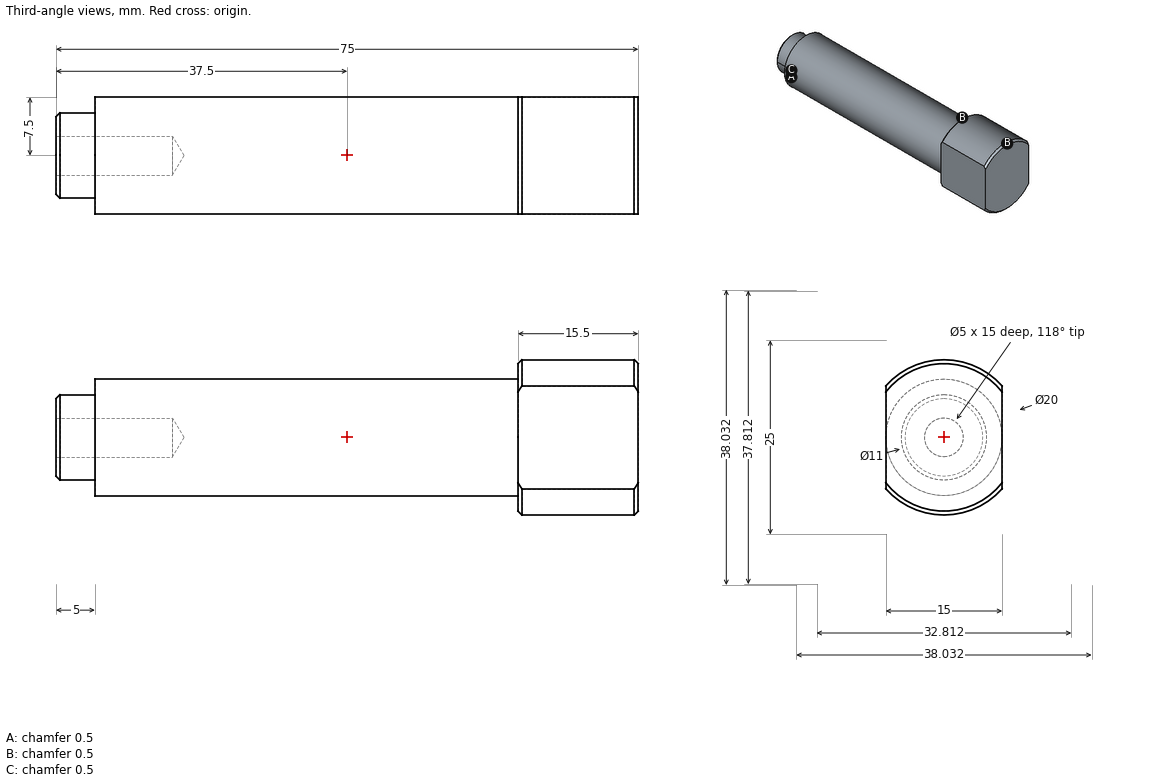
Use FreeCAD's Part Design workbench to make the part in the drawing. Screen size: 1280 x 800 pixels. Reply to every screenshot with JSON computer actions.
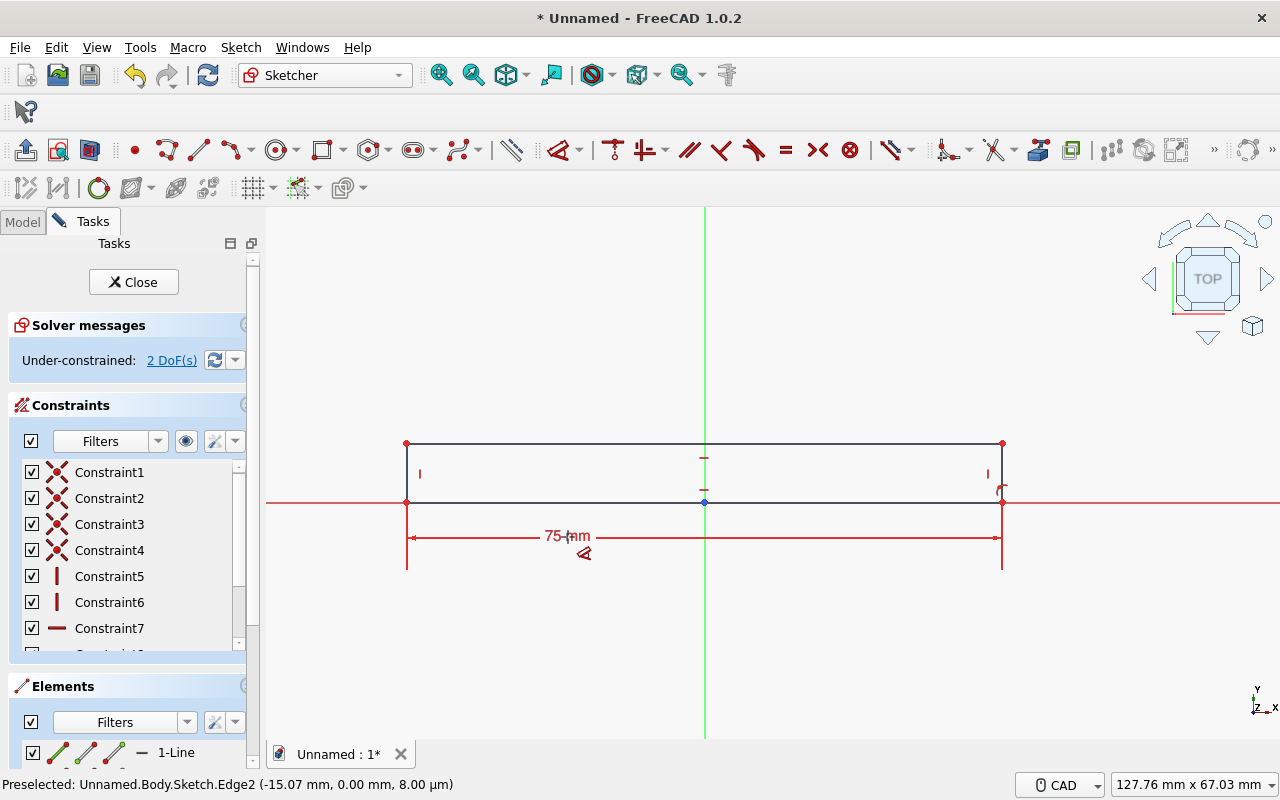
{"action": "left_click", "coordinate": [407, 462]}
{"action": "left_click", "coordinate": [373, 473]}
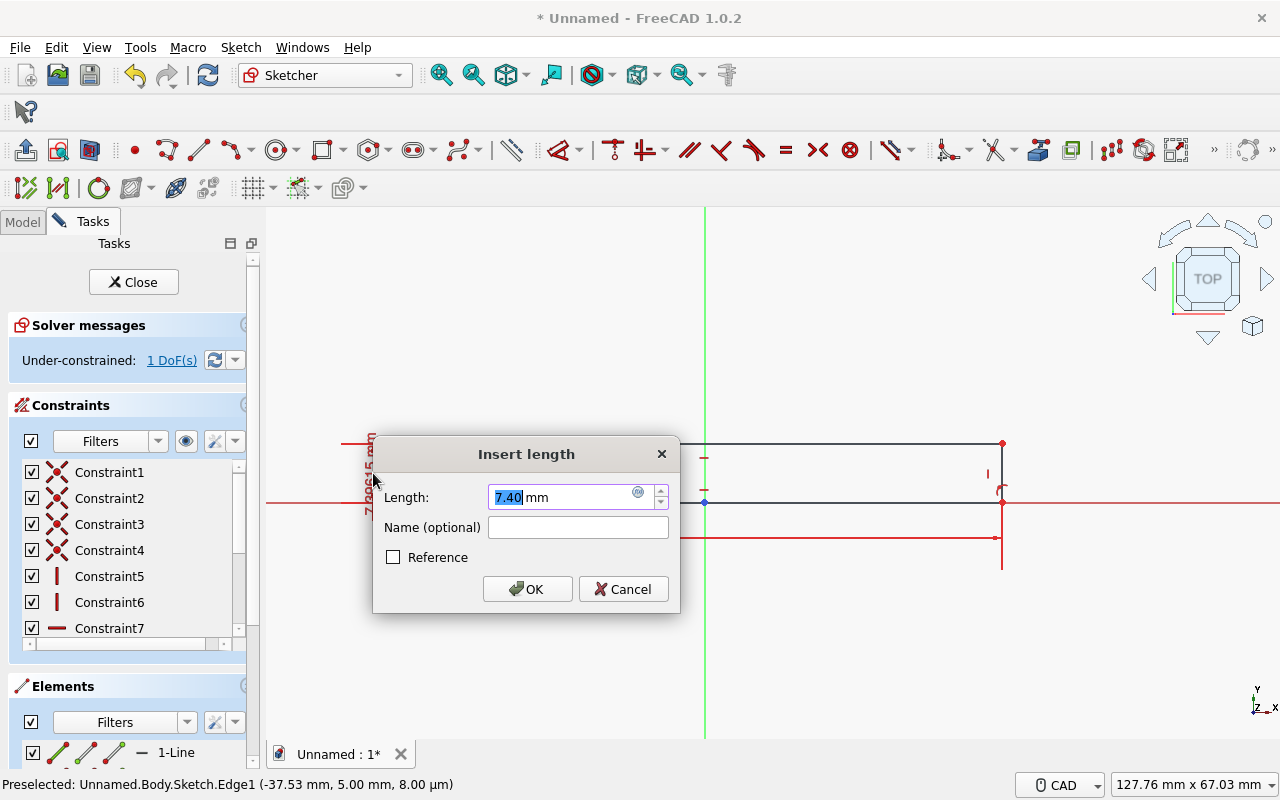
{"action": "type", "text": "7.5"}
{"action": "key", "text": "Return"}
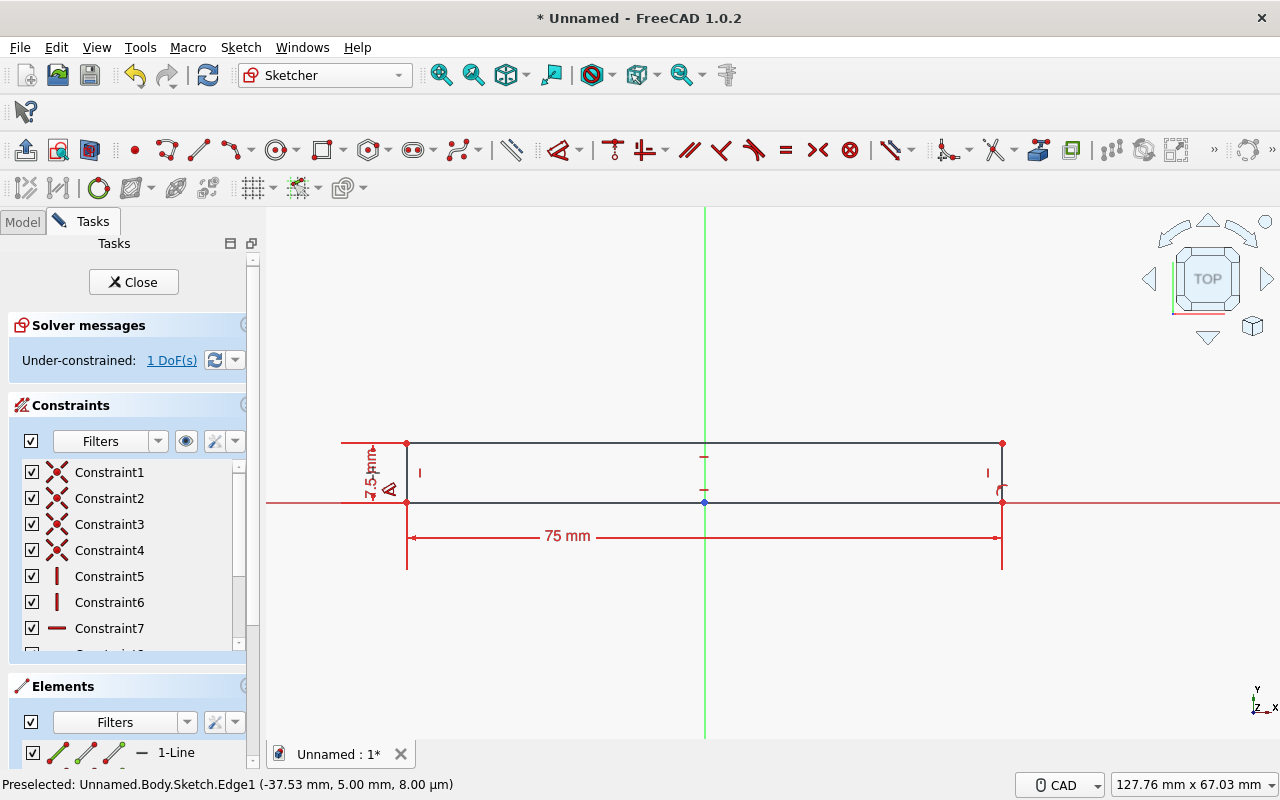
{"action": "left_click", "coordinate": [407, 443]}
{"action": "left_click", "coordinate": [487, 537]}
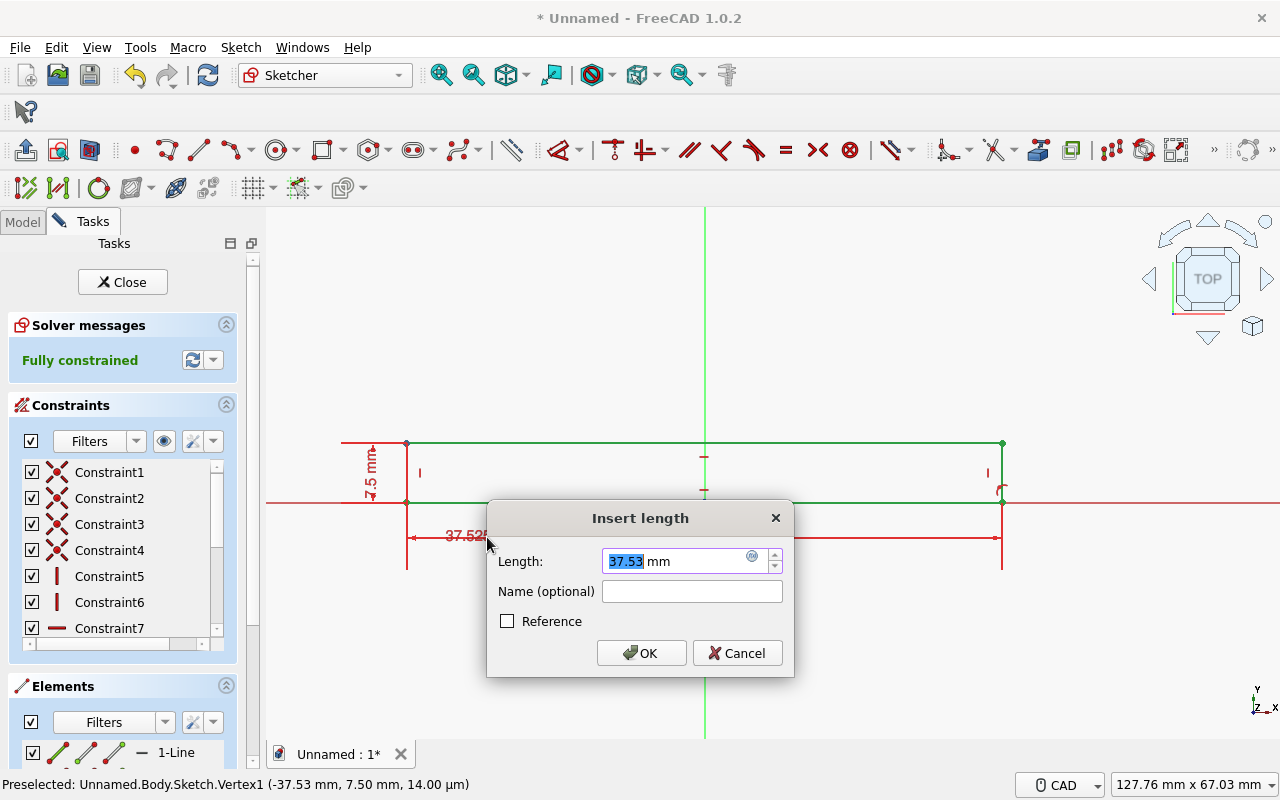
{"action": "type", "text": "37.5"}
{"action": "key", "text": "Return"}
{"action": "key", "text": "Escape"}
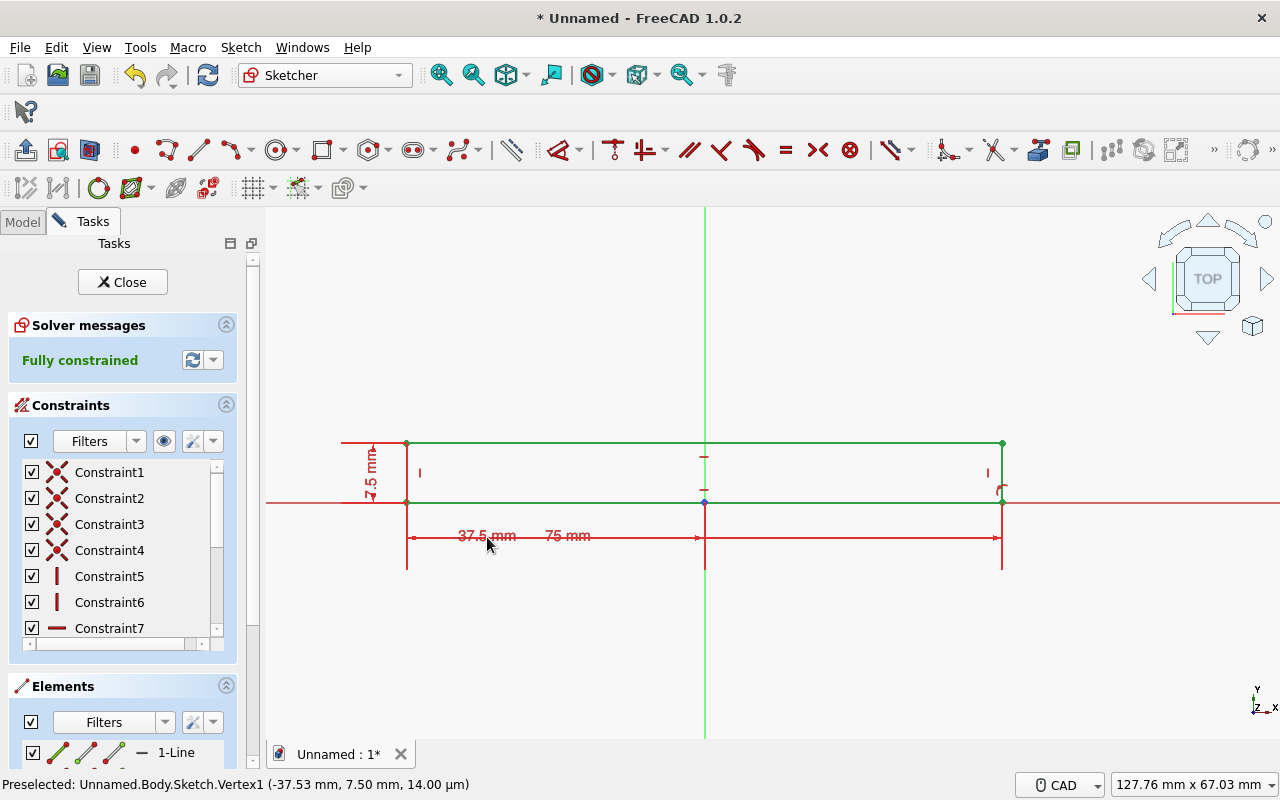
{"action": "left_click", "coordinate": [123, 282]}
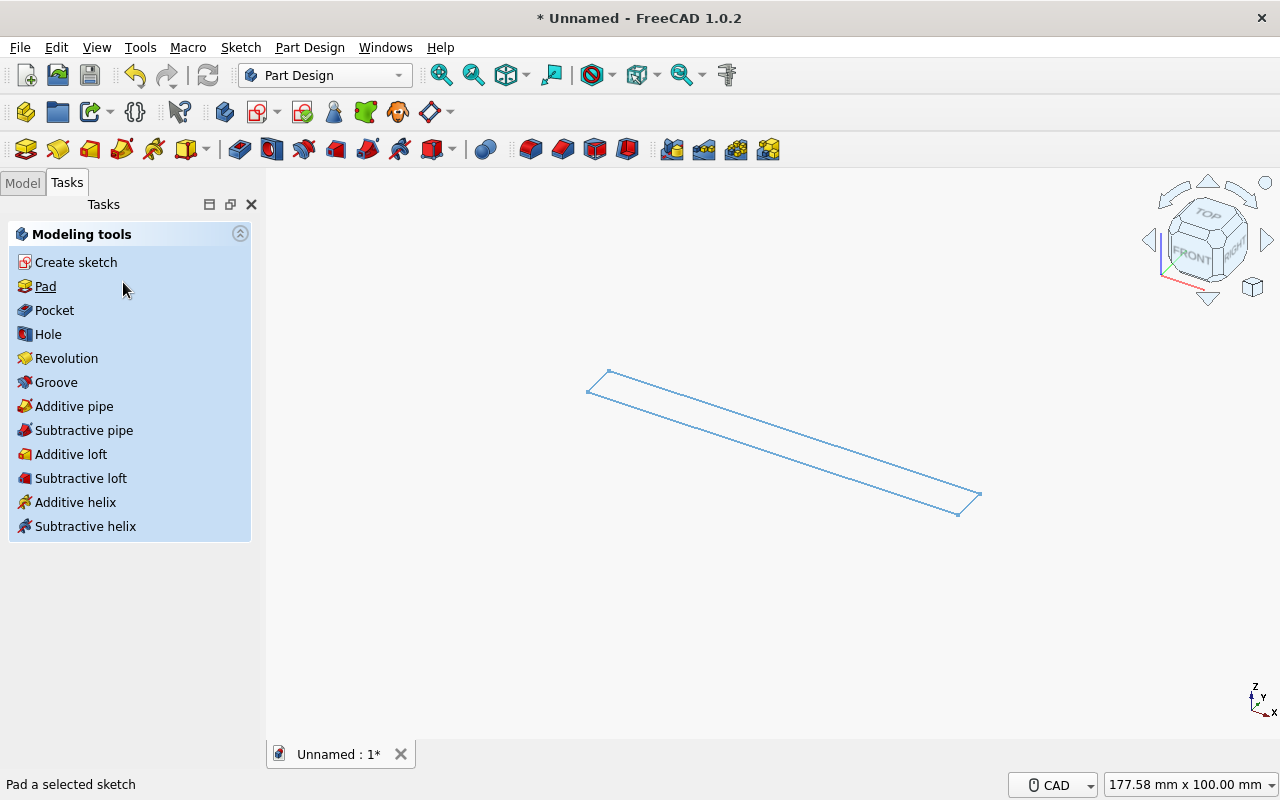
{"action": "left_click", "coordinate": [58, 150]}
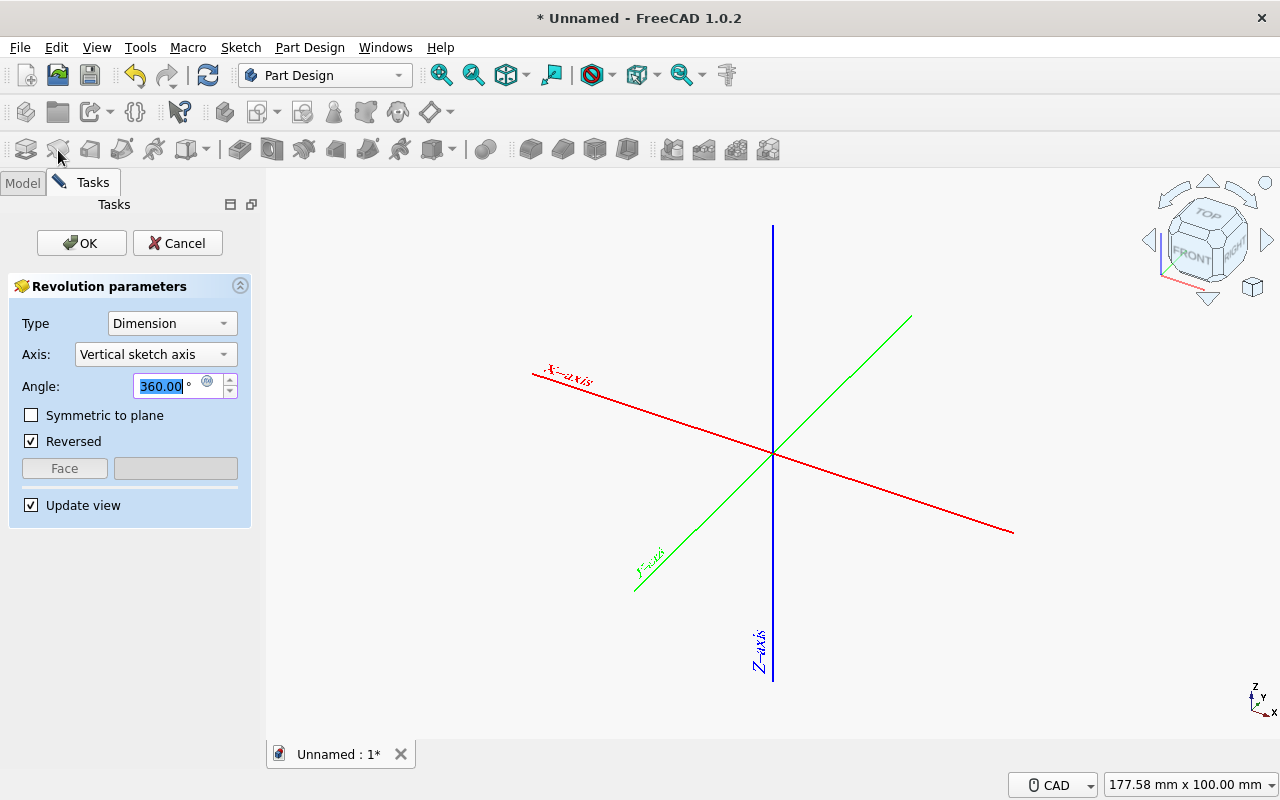
{"action": "left_click", "coordinate": [156, 354]}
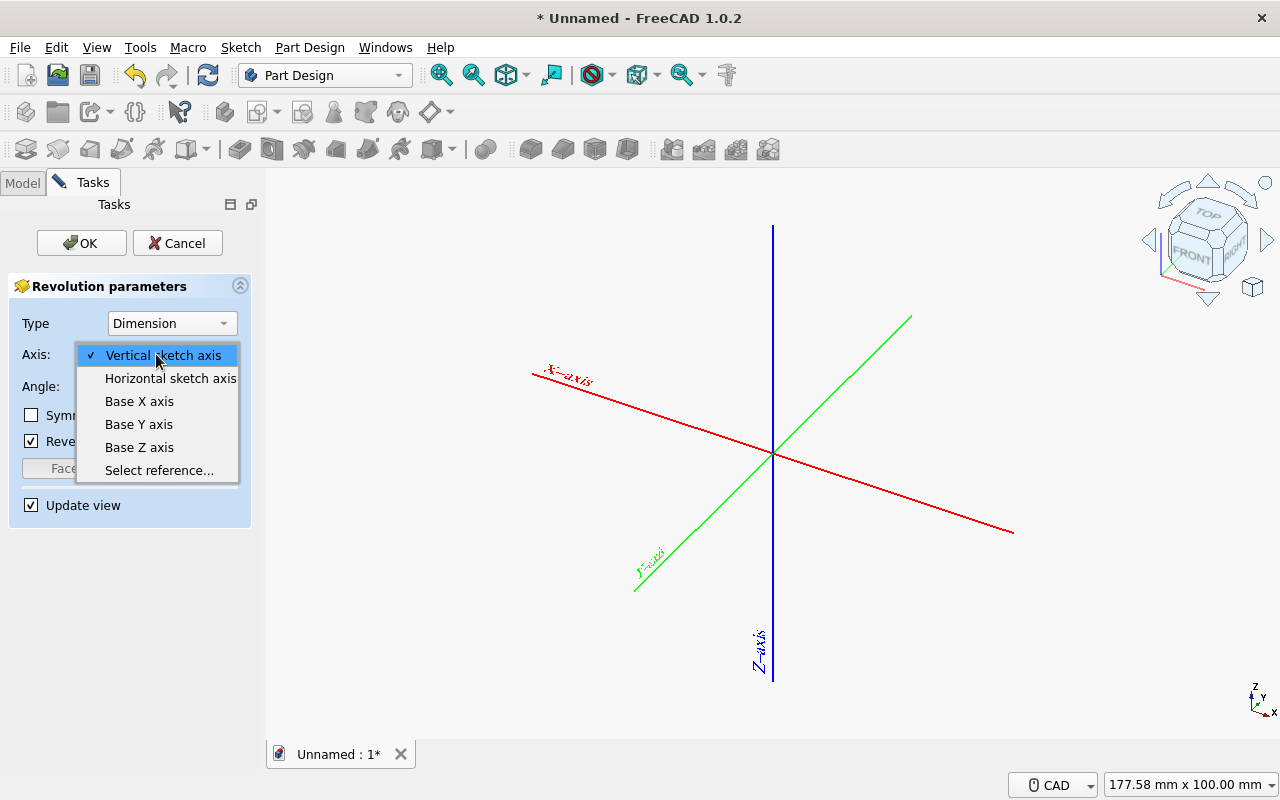
{"action": "left_click", "coordinate": [156, 378]}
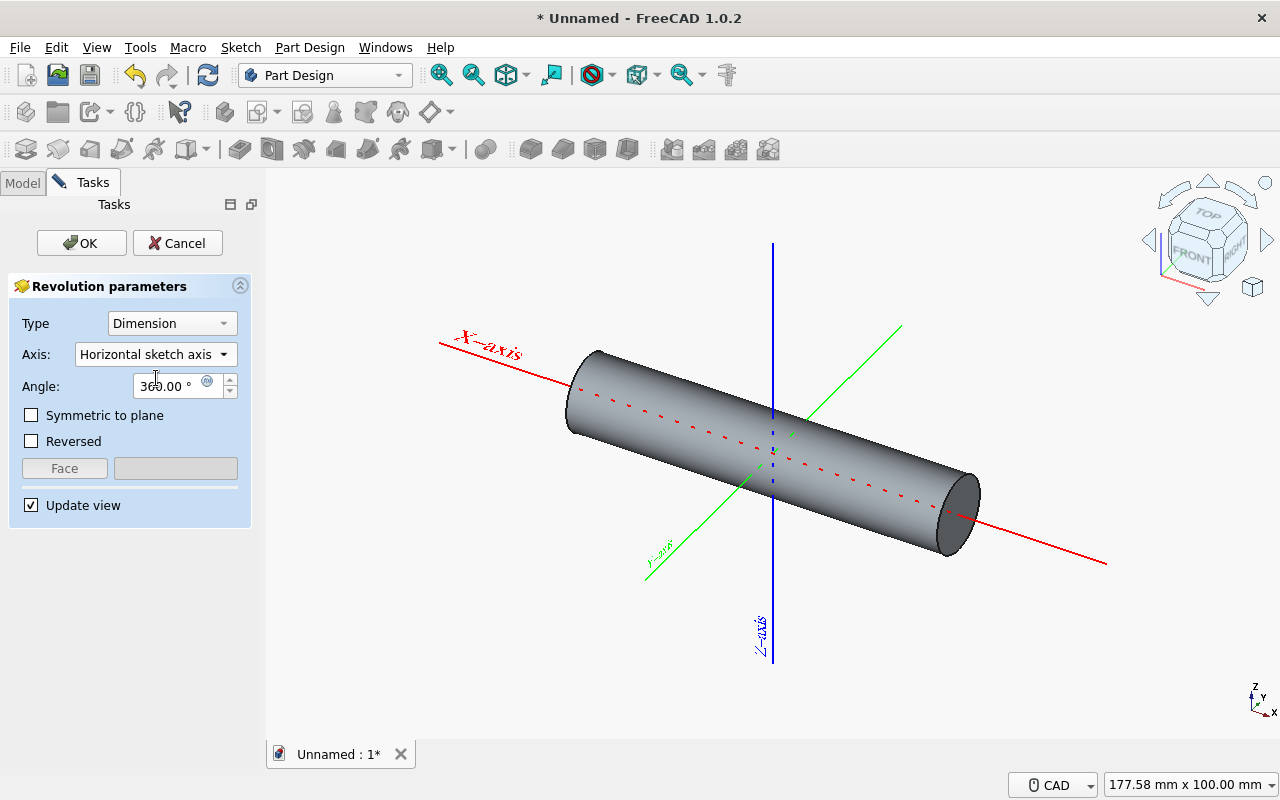
{"action": "left_click", "coordinate": [82, 243]}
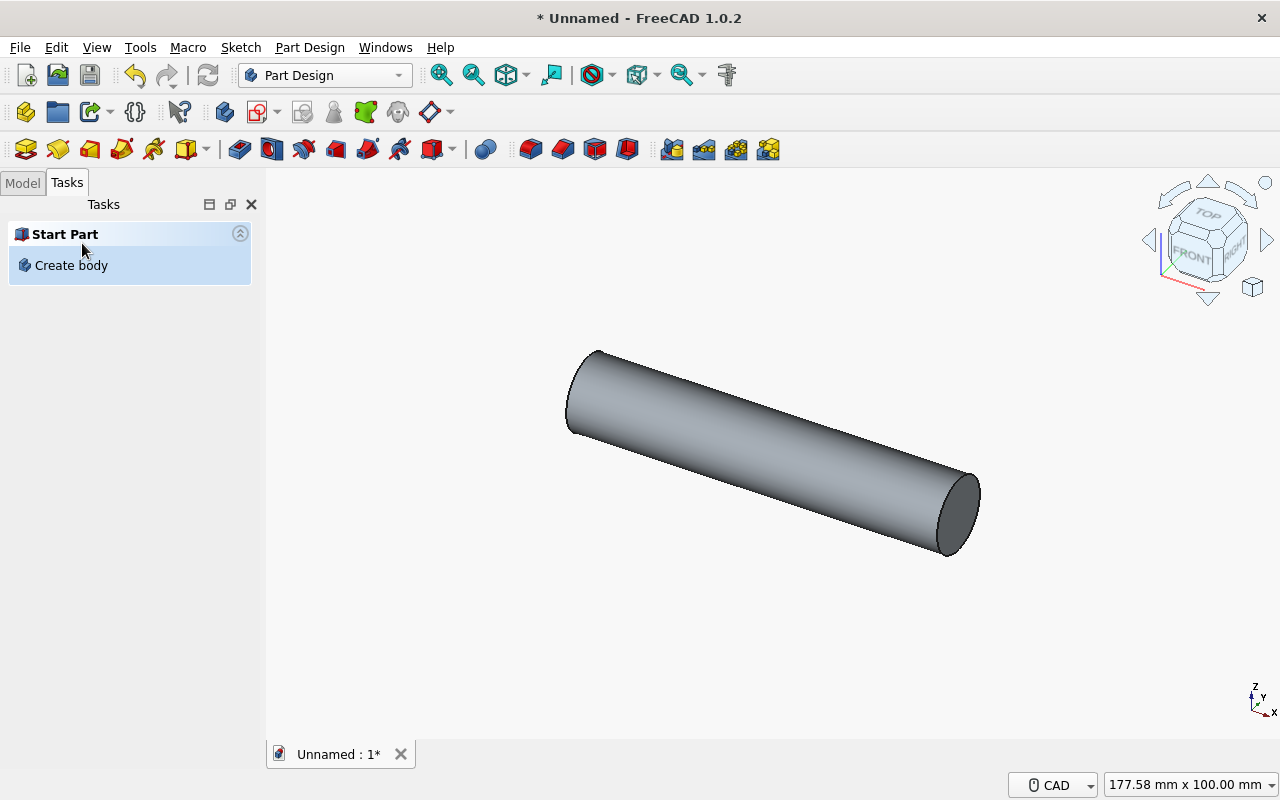
{"action": "key", "text": "v f"}